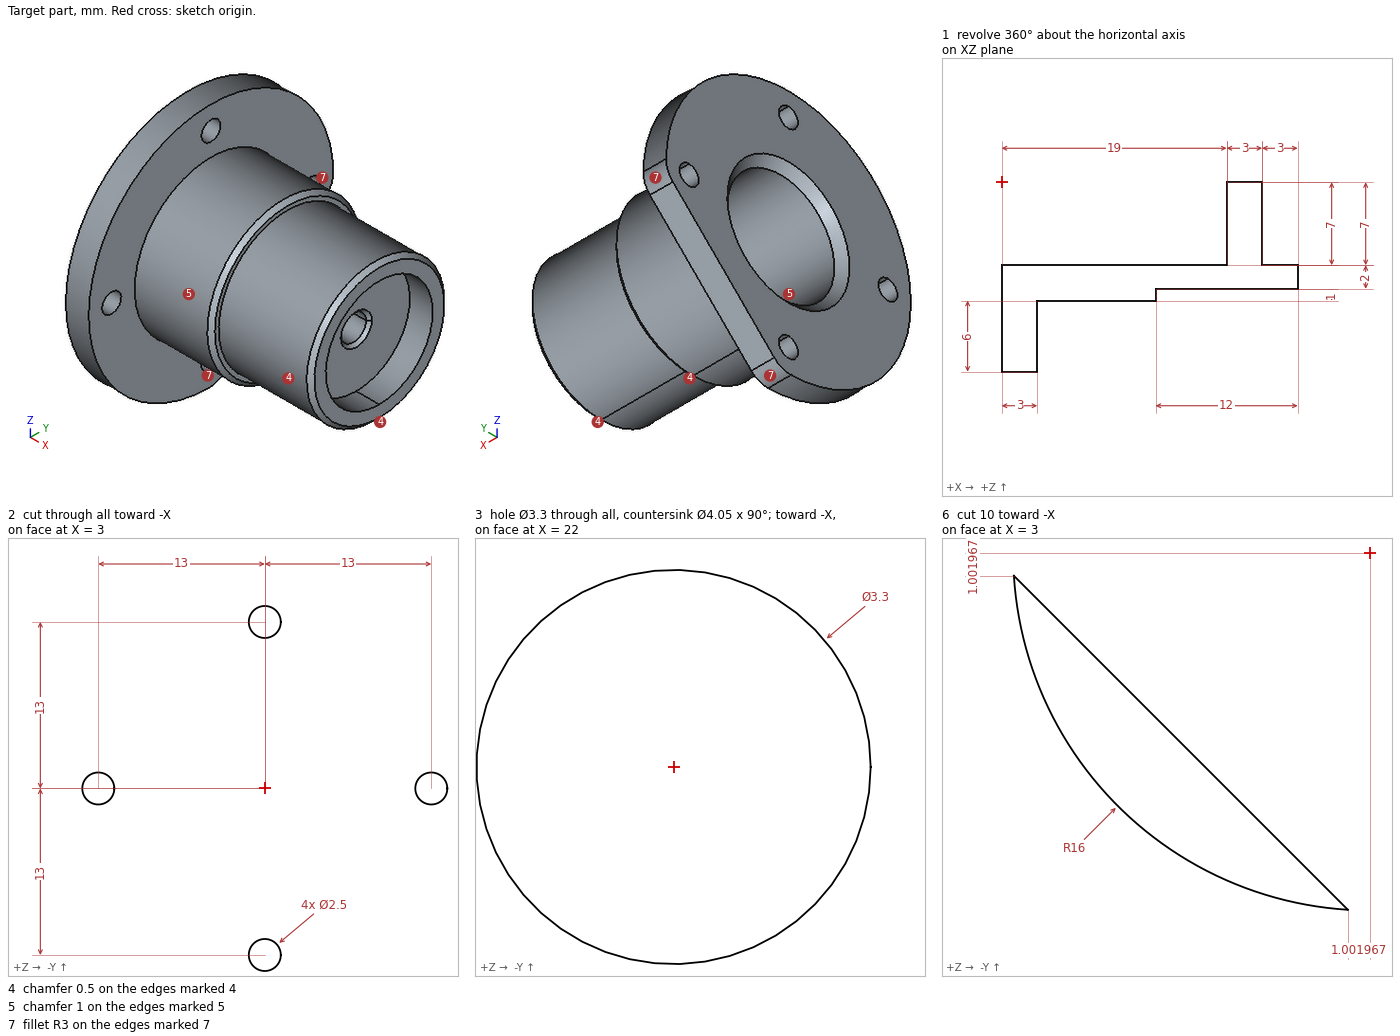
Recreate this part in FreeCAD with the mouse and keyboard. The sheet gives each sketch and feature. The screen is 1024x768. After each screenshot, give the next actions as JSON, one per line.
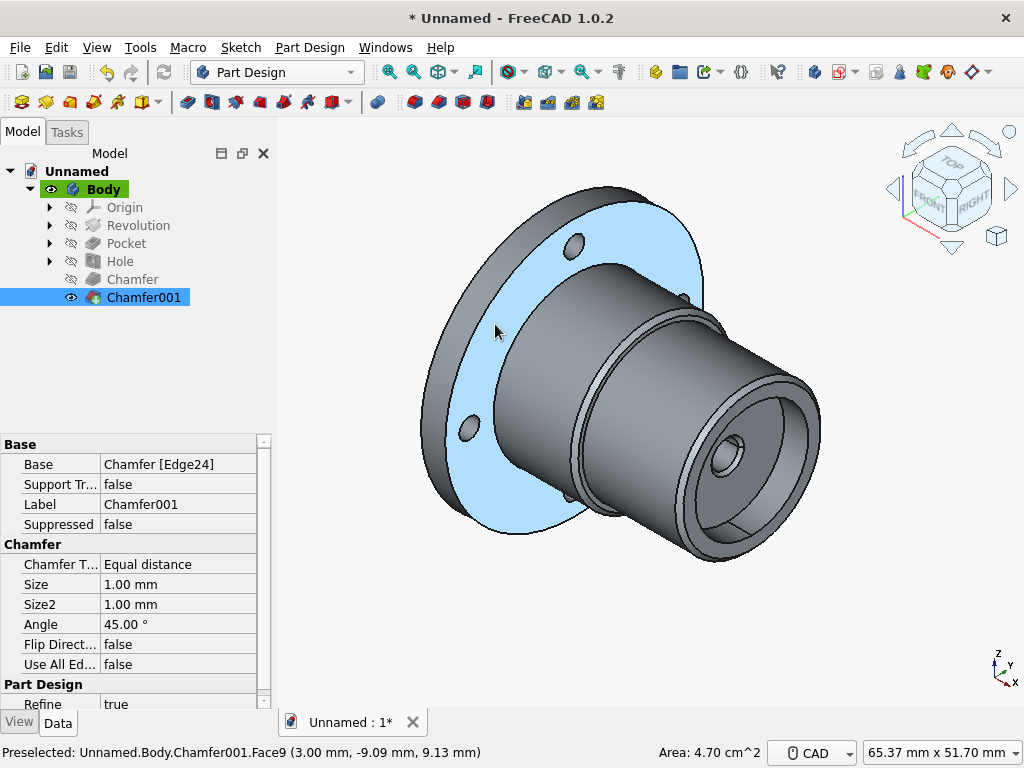
{"action": "left_click", "coordinate": [840, 72]}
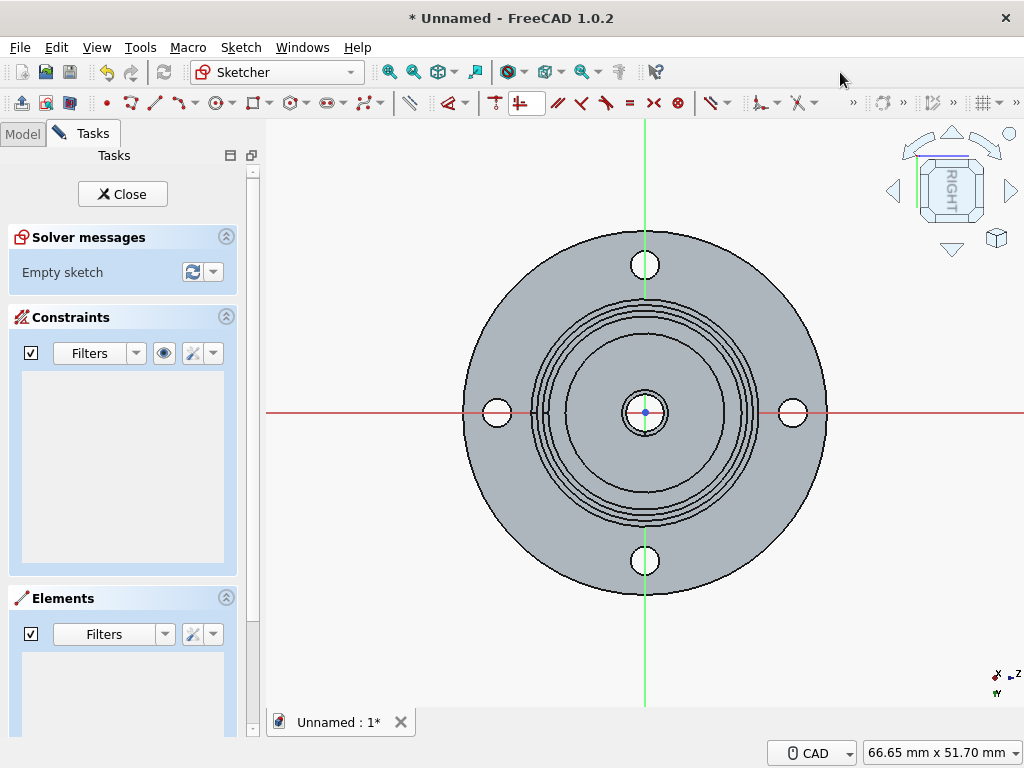
{"action": "left_click", "coordinate": [70, 104]}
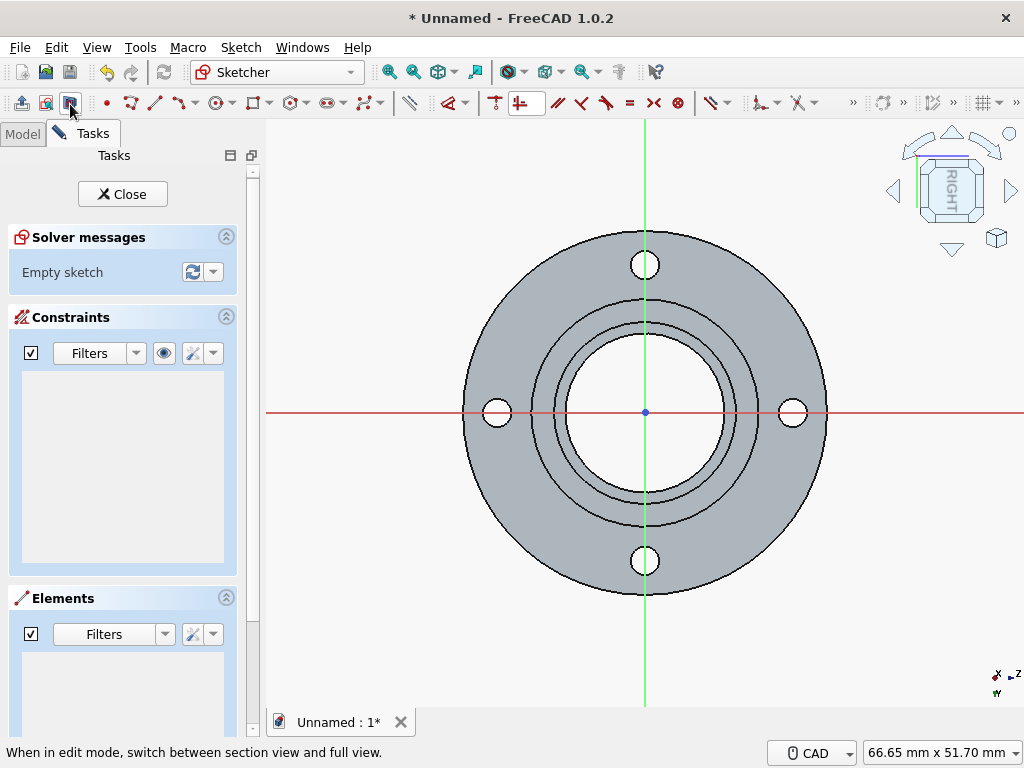
{"action": "scroll", "coordinate": [536, 578], "scroll_direction": "up", "scroll_amount": 4}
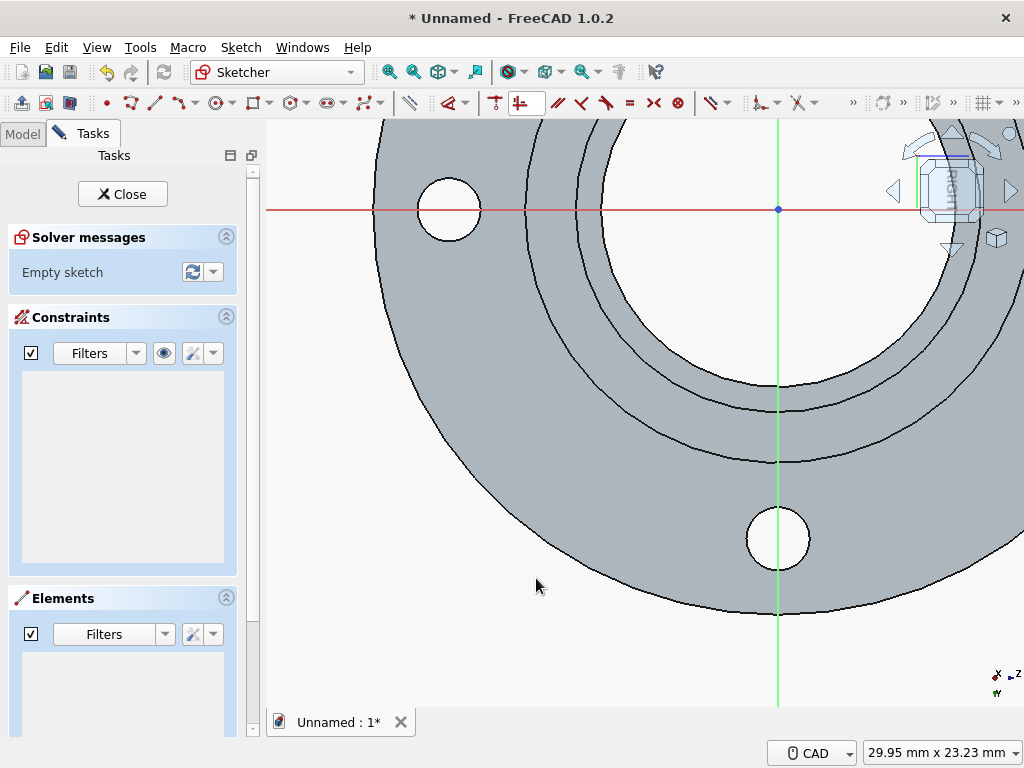
{"action": "left_click", "coordinate": [156, 104]}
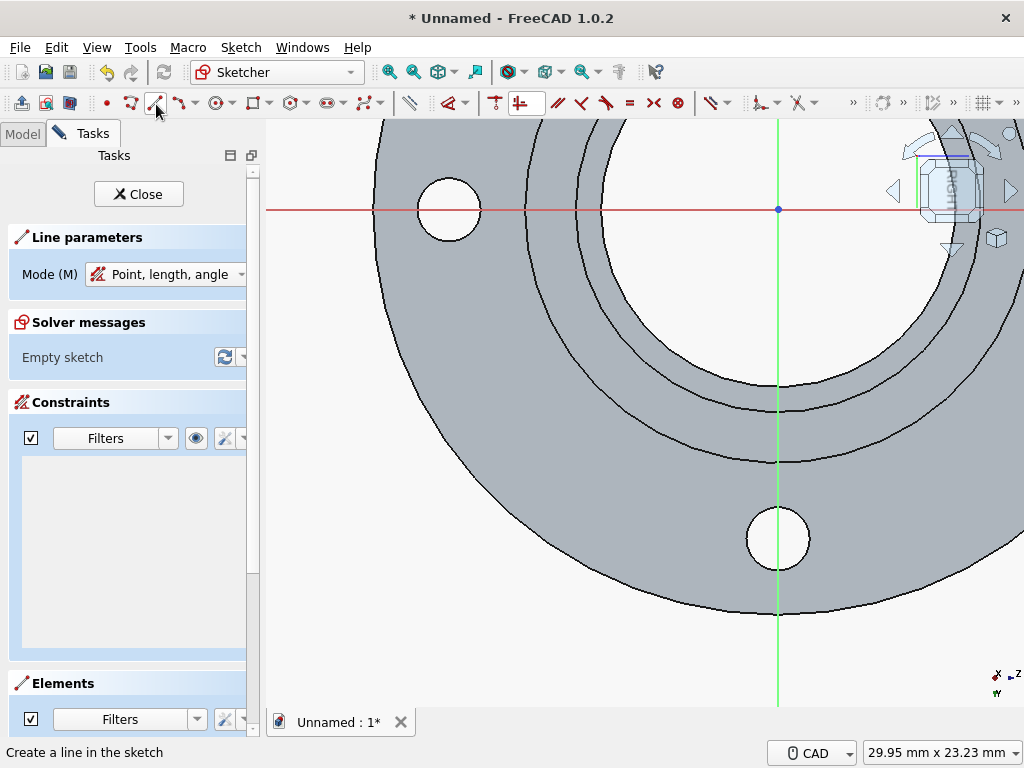
{"action": "left_click", "coordinate": [753, 614]}
{"action": "left_click", "coordinate": [374, 235]}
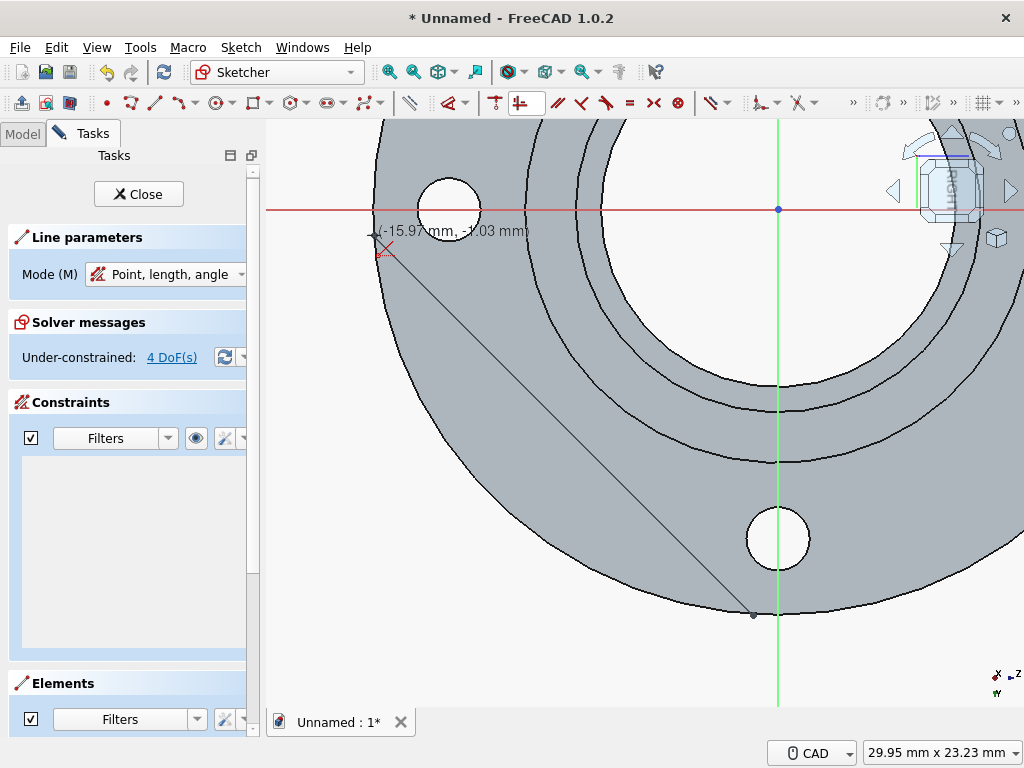
{"action": "left_click", "coordinate": [180, 104]}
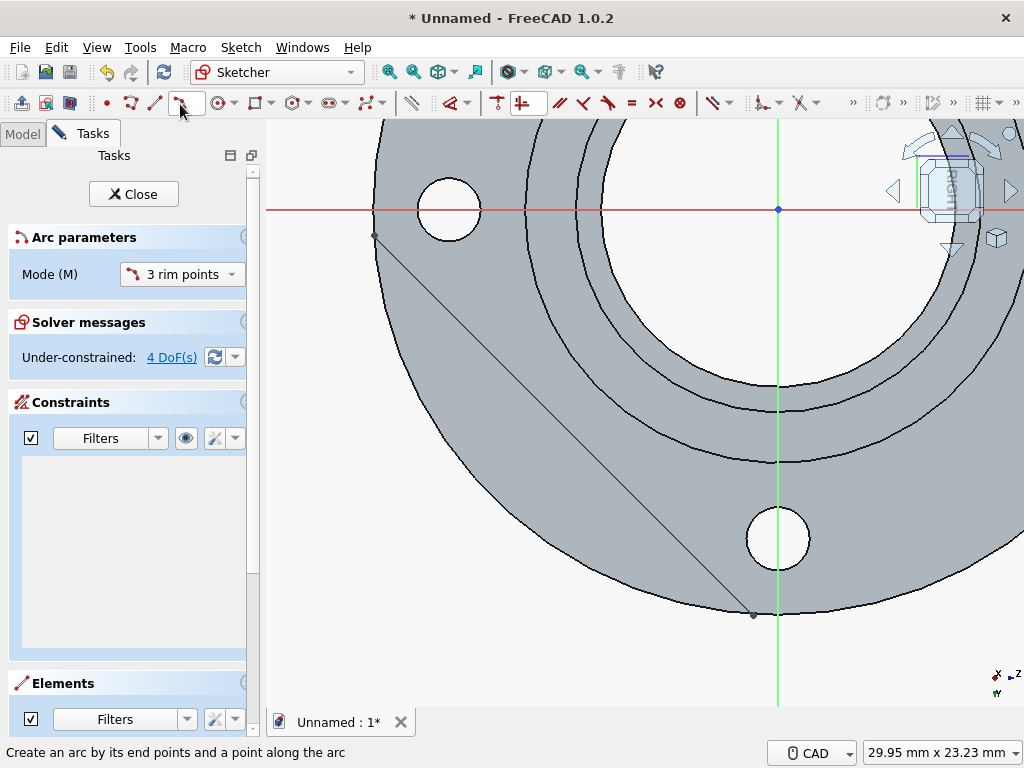
{"action": "left_click", "coordinate": [374, 236]}
{"action": "left_click", "coordinate": [753, 615]}
{"action": "left_click", "coordinate": [492, 496]}
{"action": "key", "text": "Escape"}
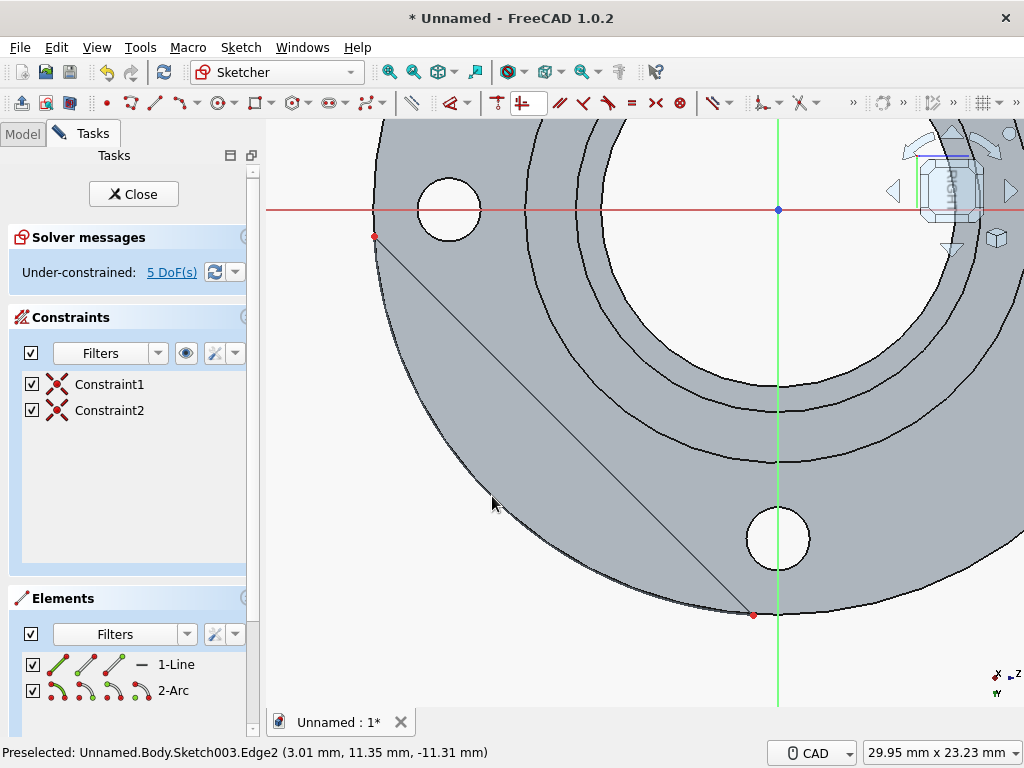
{"action": "left_click_drag", "start_coordinate": [768, 200], "coordinate": [789, 220]}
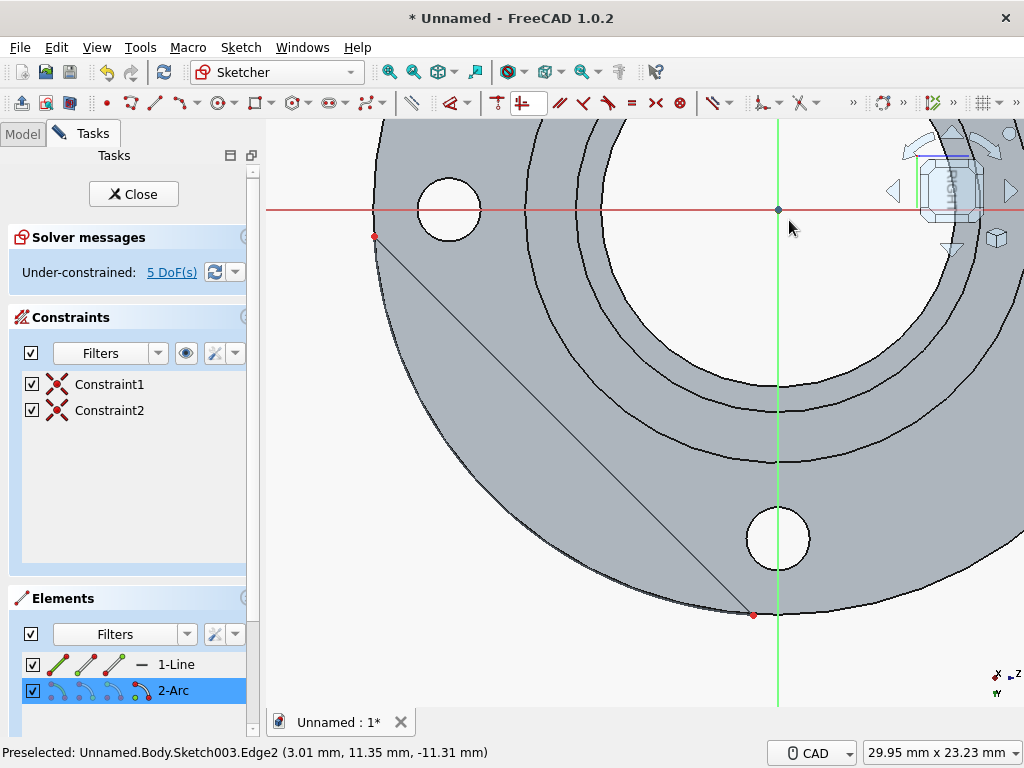
{"action": "left_click", "coordinate": [498, 104]}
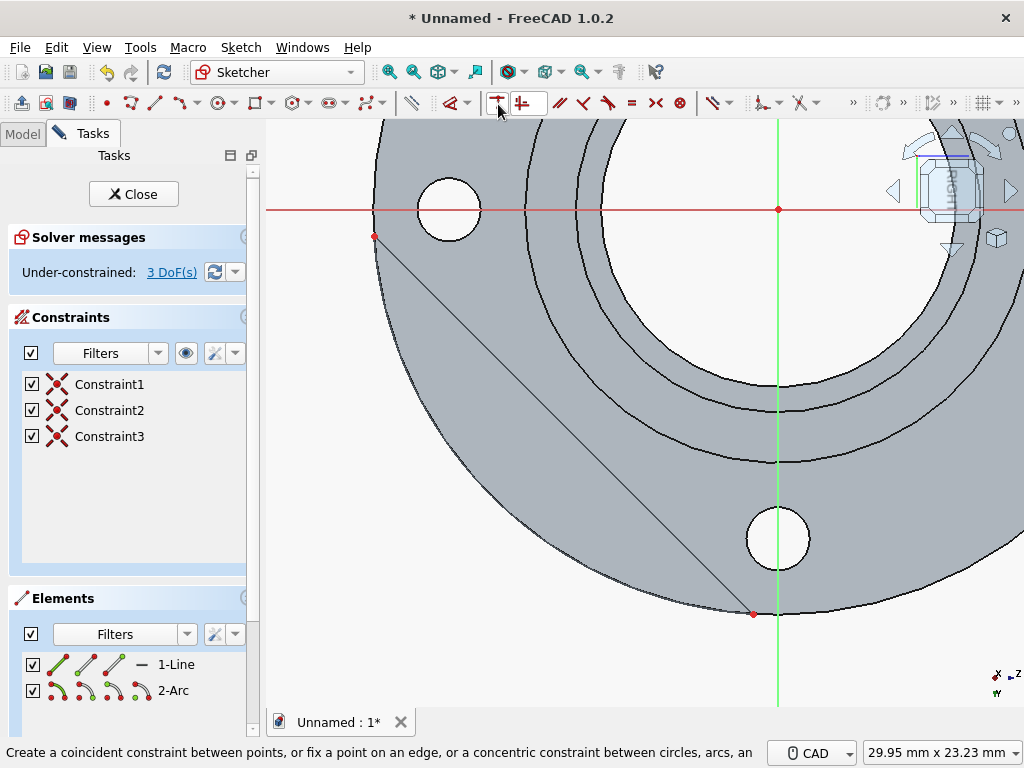
{"action": "left_click", "coordinate": [450, 104]}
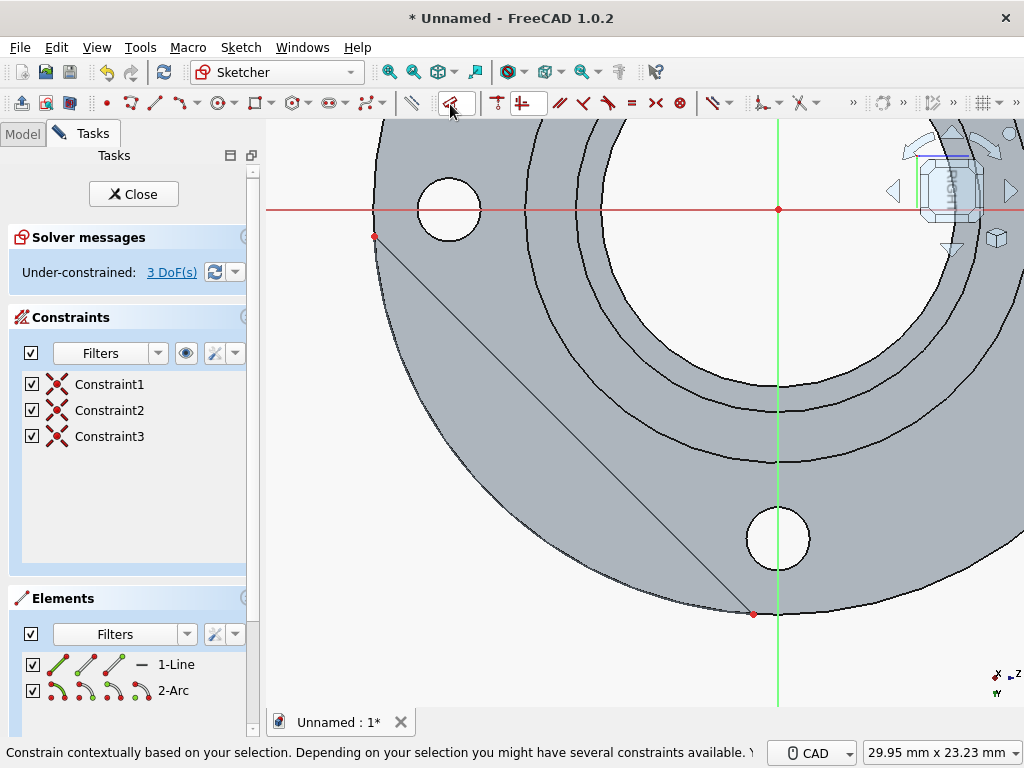
{"action": "left_click", "coordinate": [422, 403]}
{"action": "left_click", "coordinate": [394, 418]}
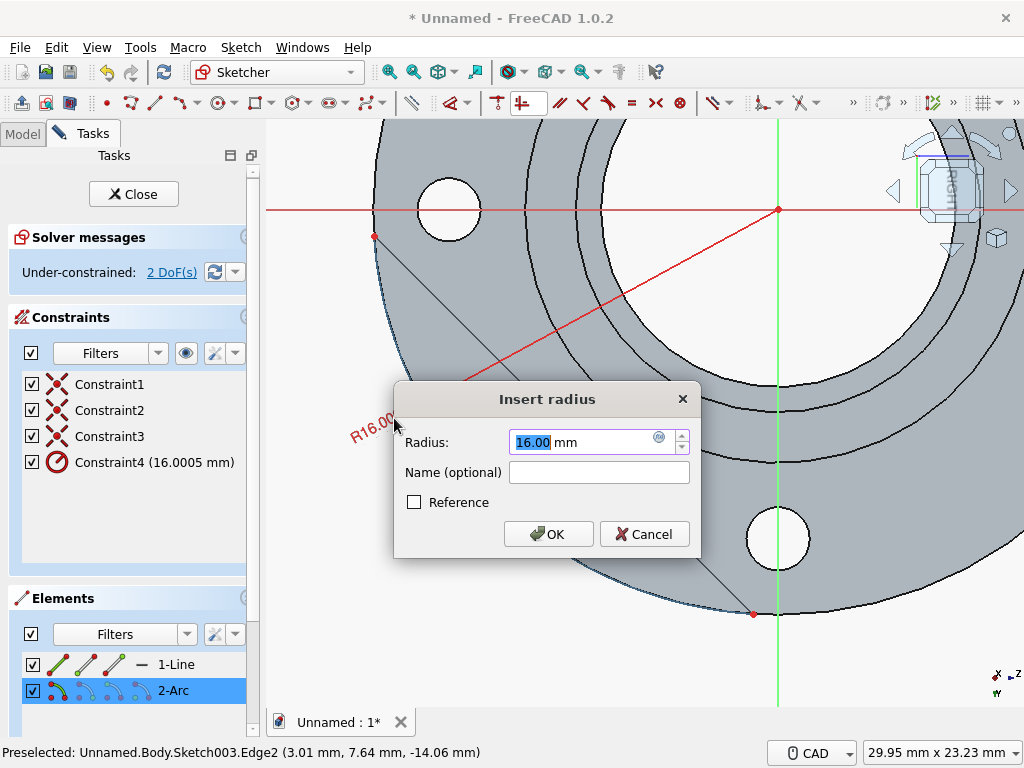
{"action": "type", "text": "16"}
{"action": "key", "text": "Return"}